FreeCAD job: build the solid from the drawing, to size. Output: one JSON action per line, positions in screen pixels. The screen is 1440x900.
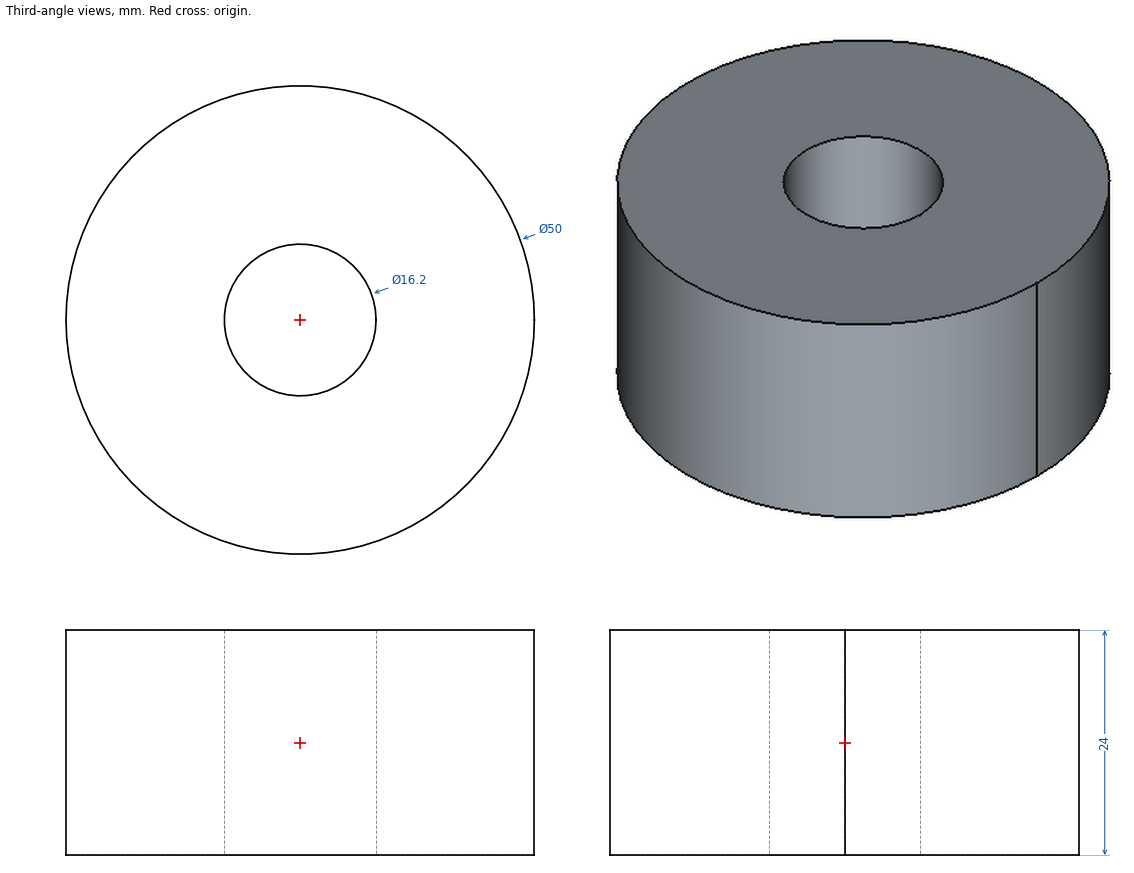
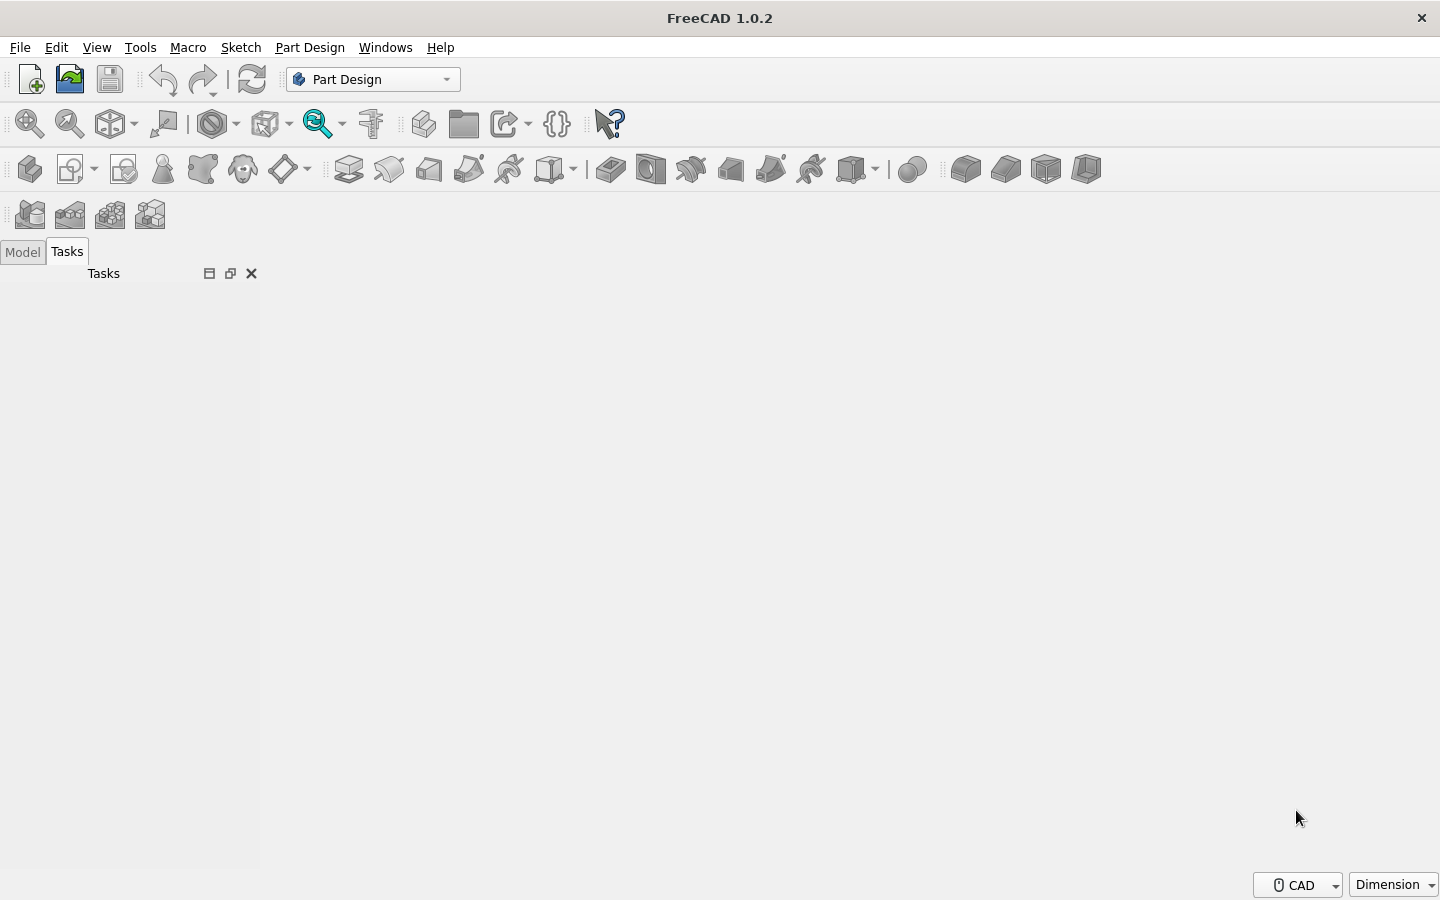
{"action": "left_click", "coordinate": [30, 80]}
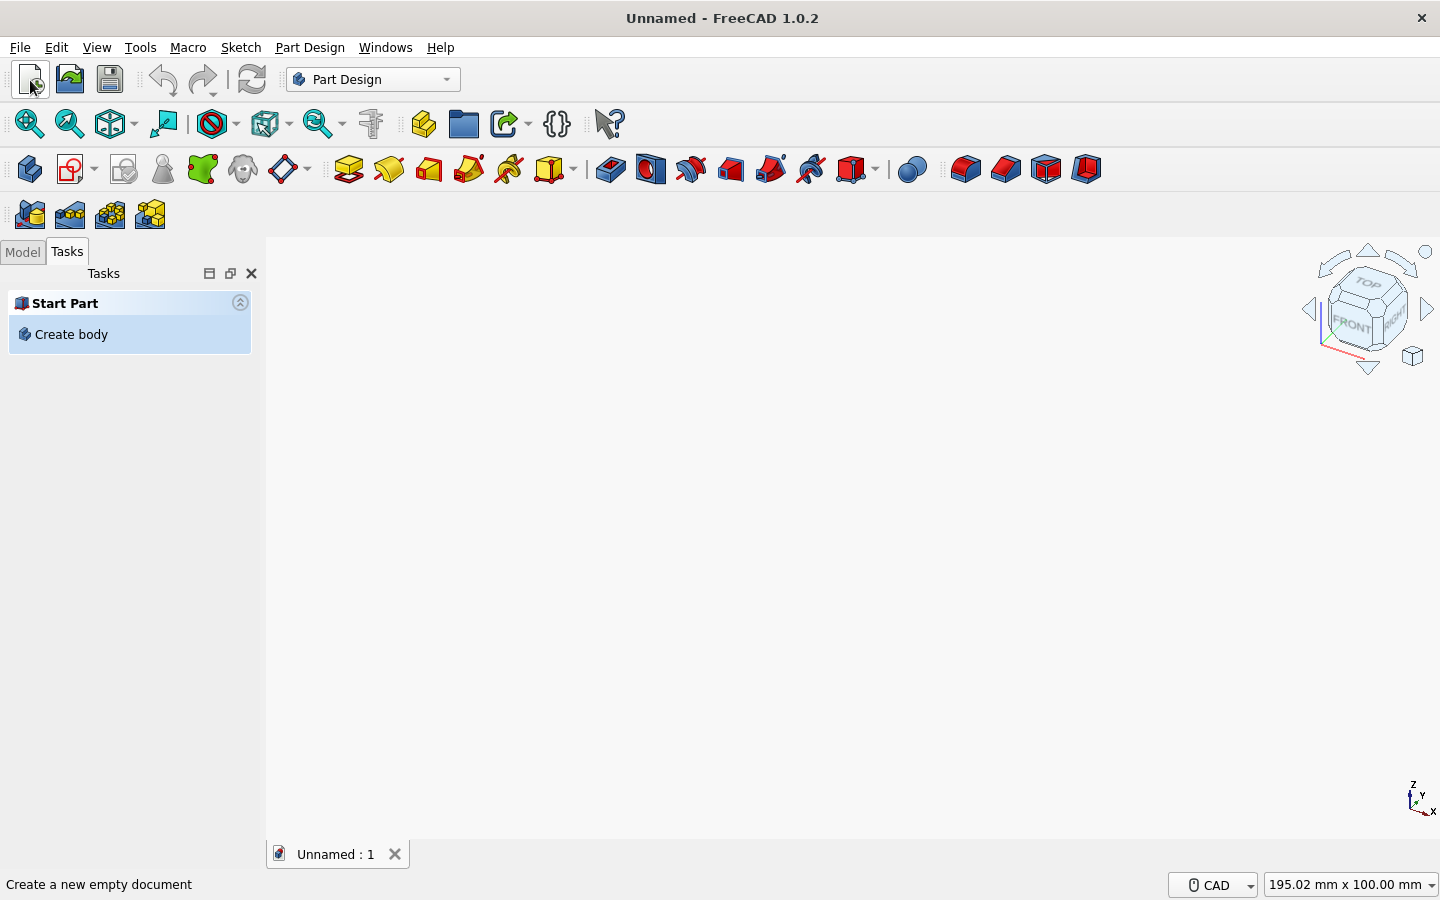
{"action": "left_click", "coordinate": [70, 170]}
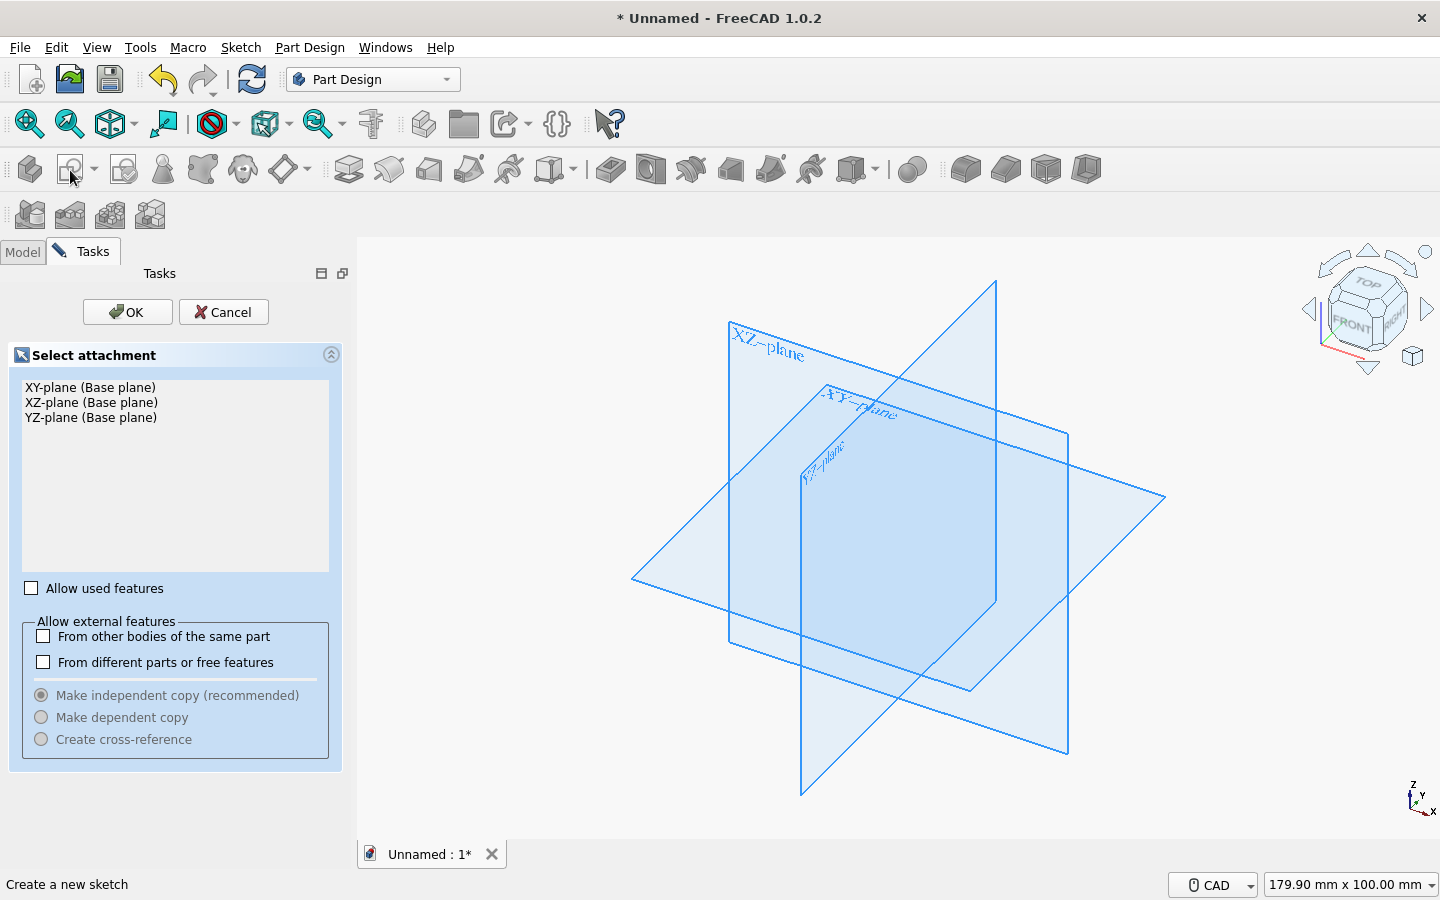
{"action": "left_click", "coordinate": [82, 388]}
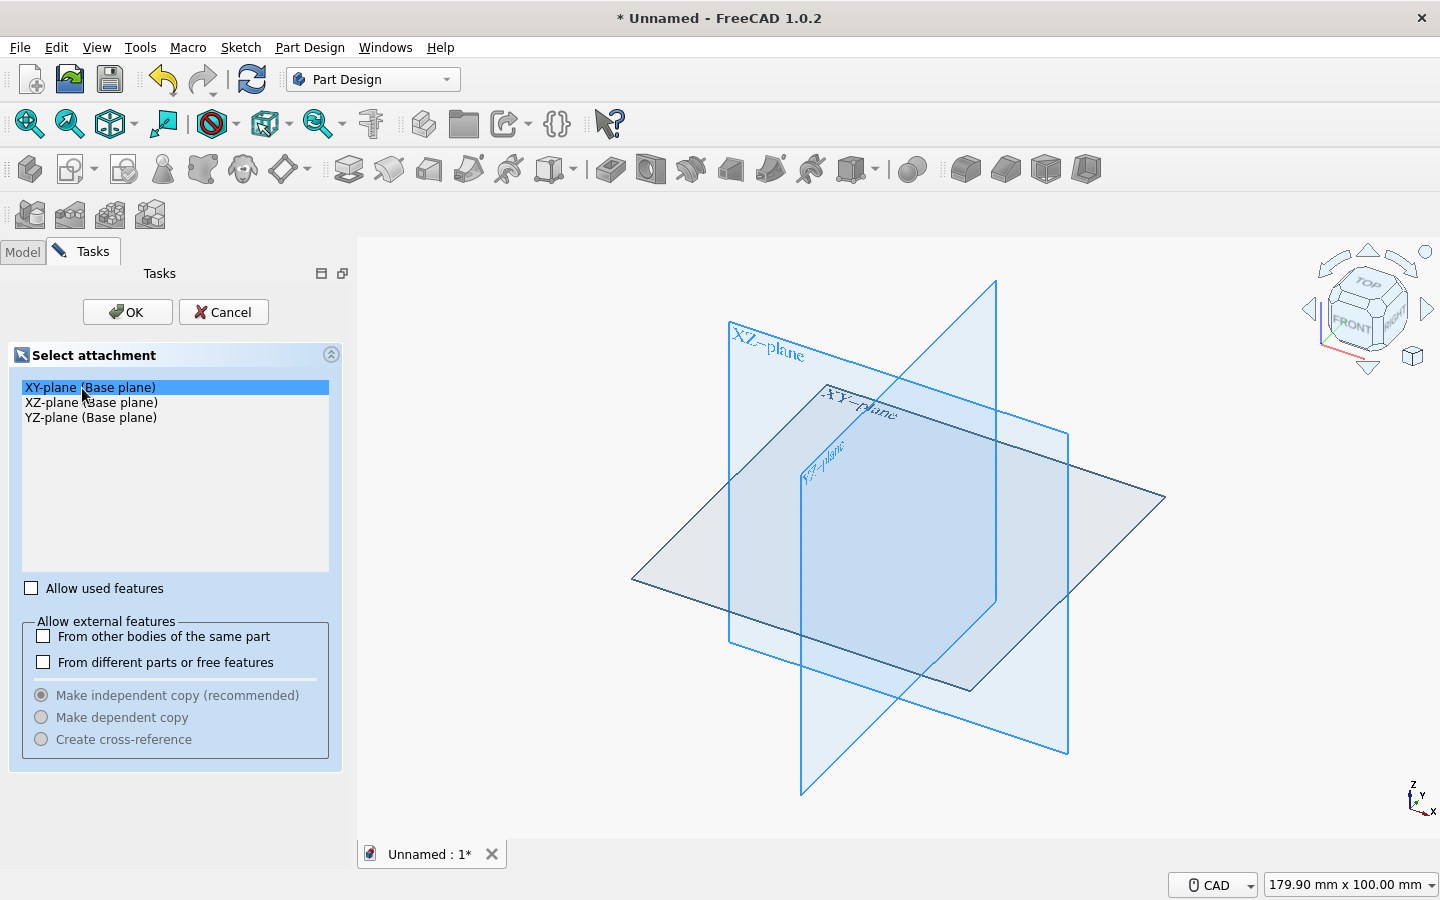
{"action": "left_click", "coordinate": [128, 312]}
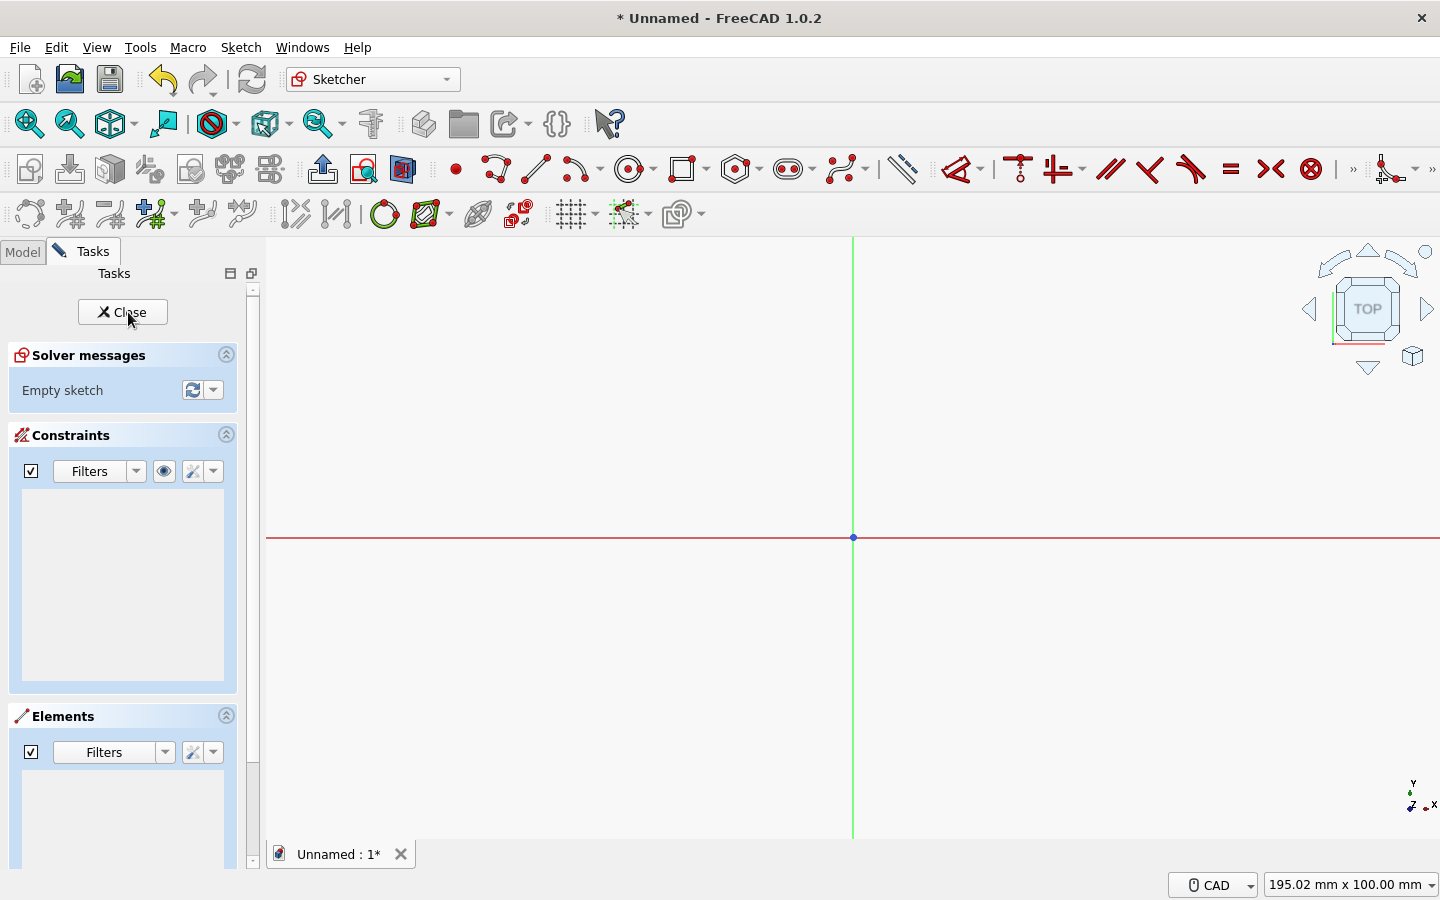
{"action": "left_click", "coordinate": [630, 170]}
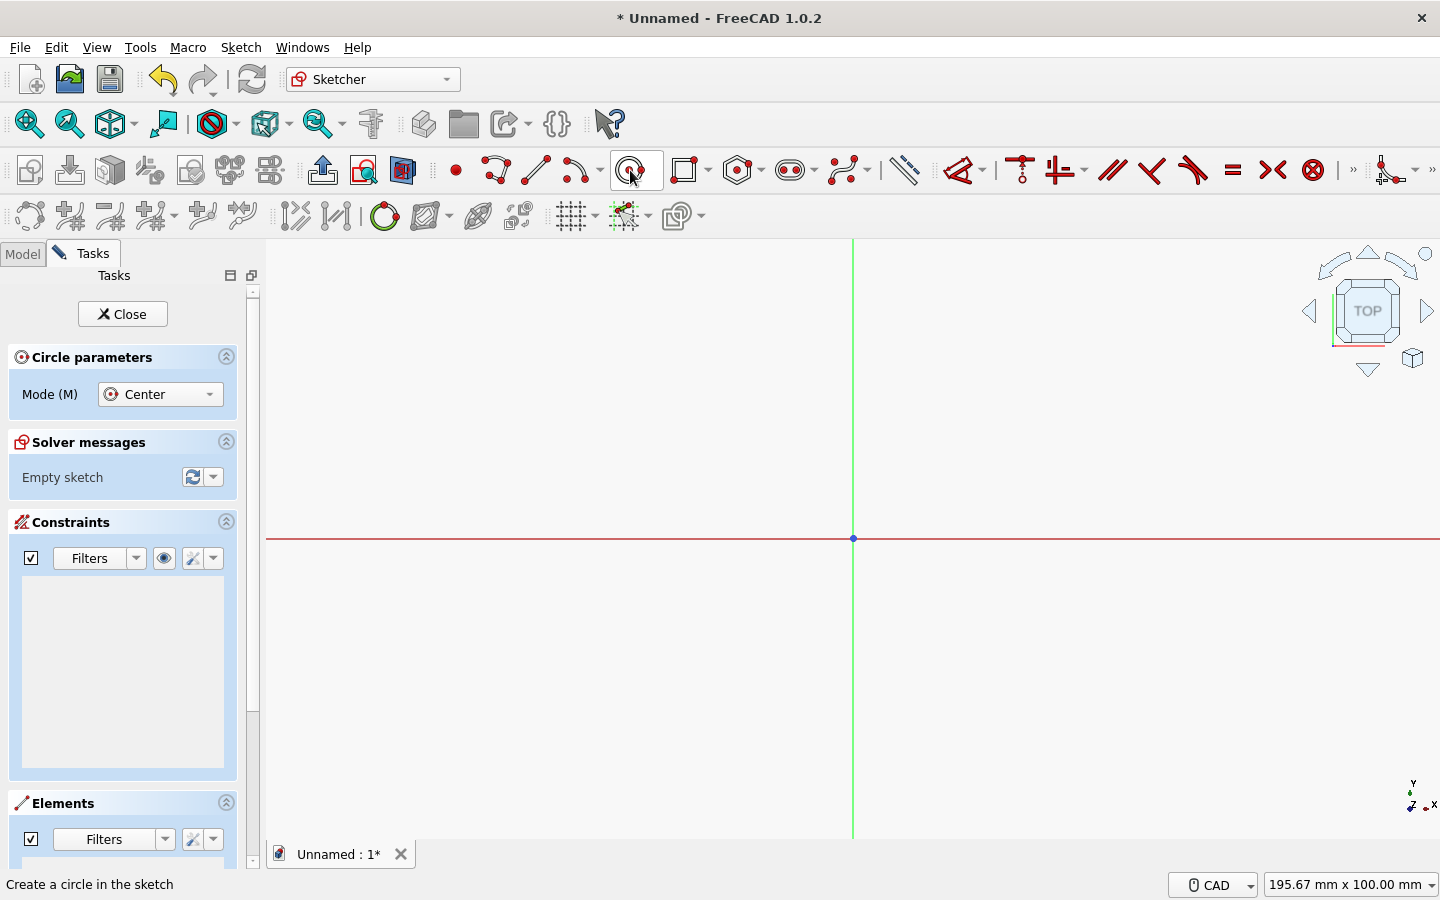
{"action": "left_click", "coordinate": [853, 539]}
{"action": "mouse_move", "coordinate": [959, 433]}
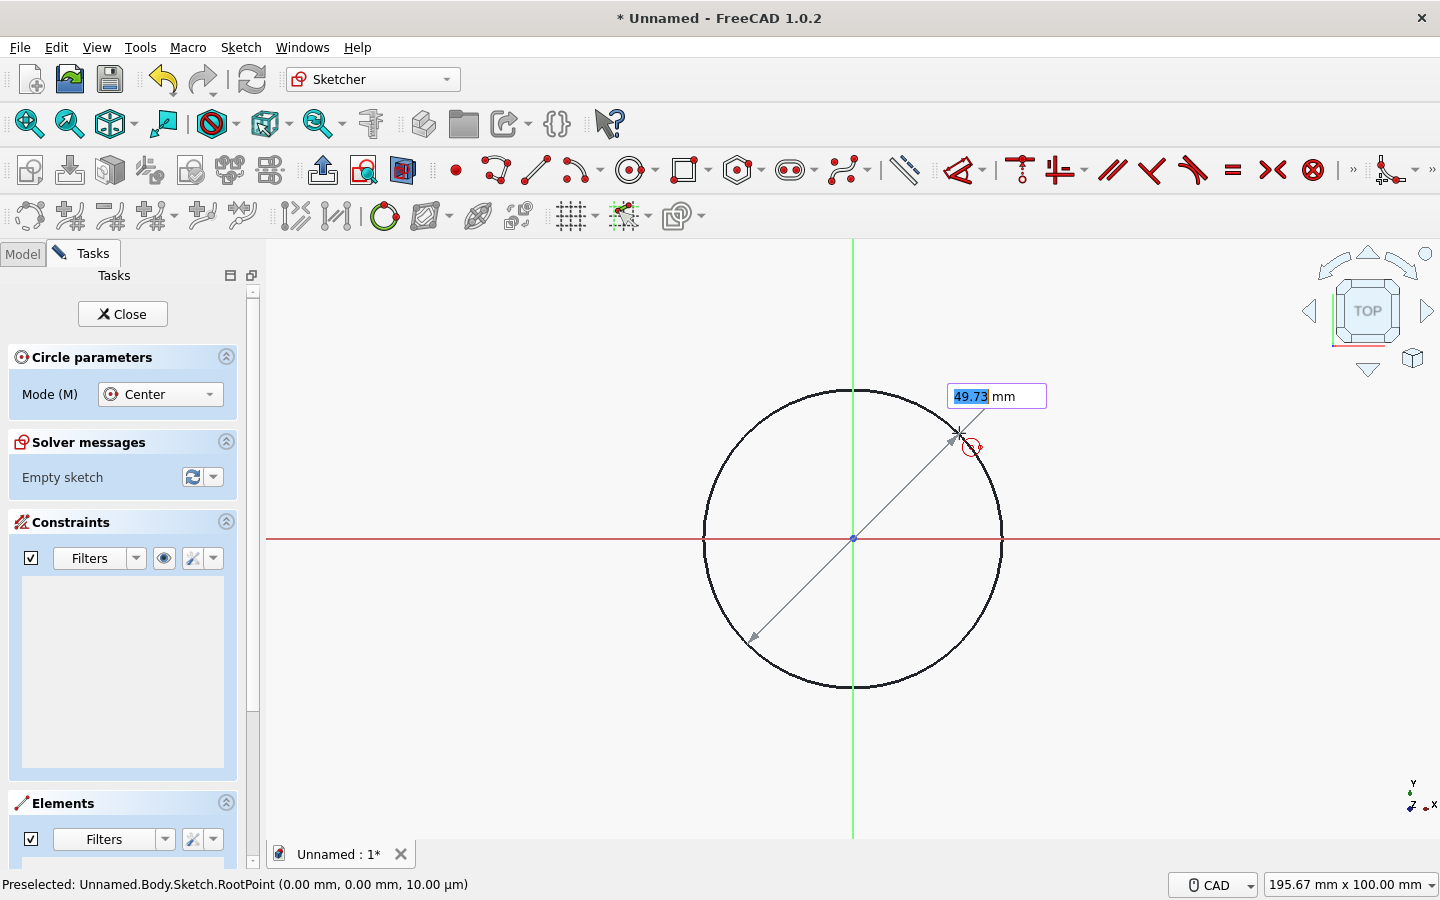
{"action": "type", "text": "50"}
{"action": "key", "text": "Return"}